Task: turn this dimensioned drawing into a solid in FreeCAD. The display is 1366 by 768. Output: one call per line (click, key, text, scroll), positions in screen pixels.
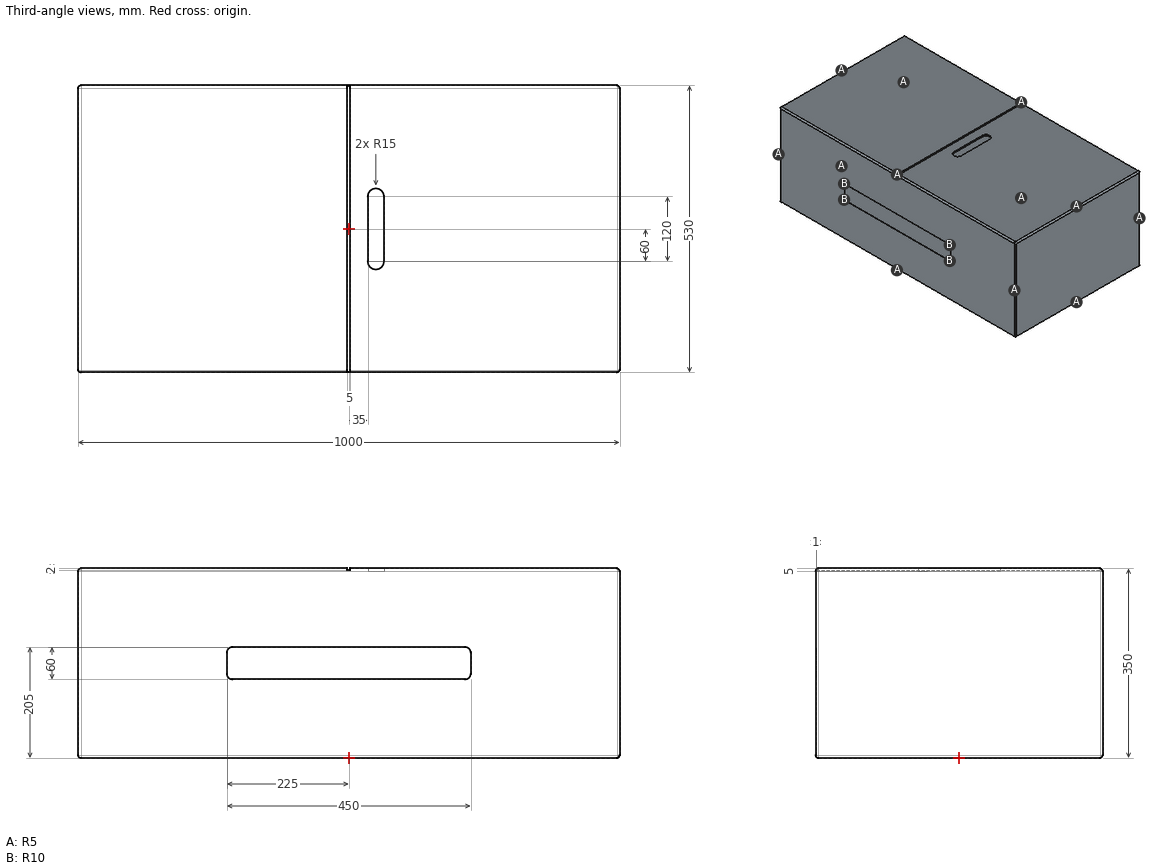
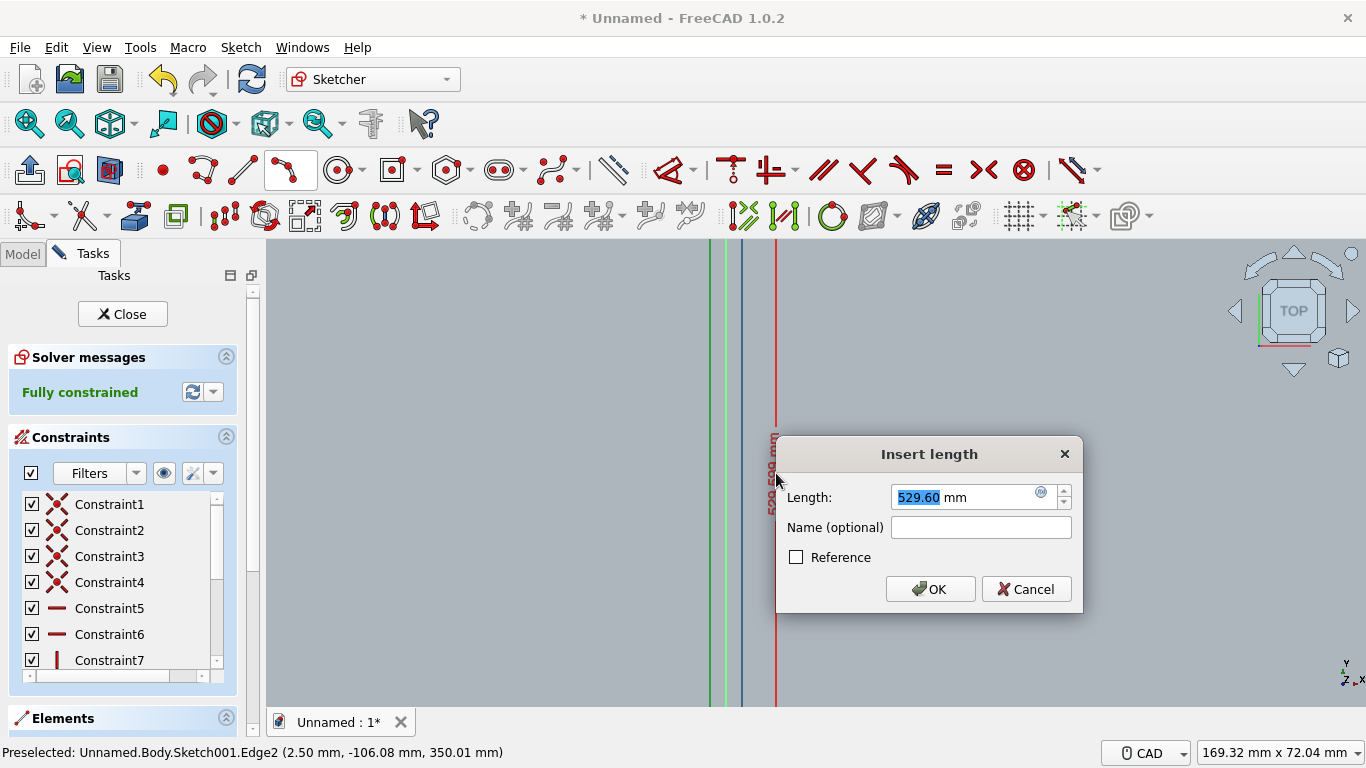
text(530)
key(Return)
key(Escape)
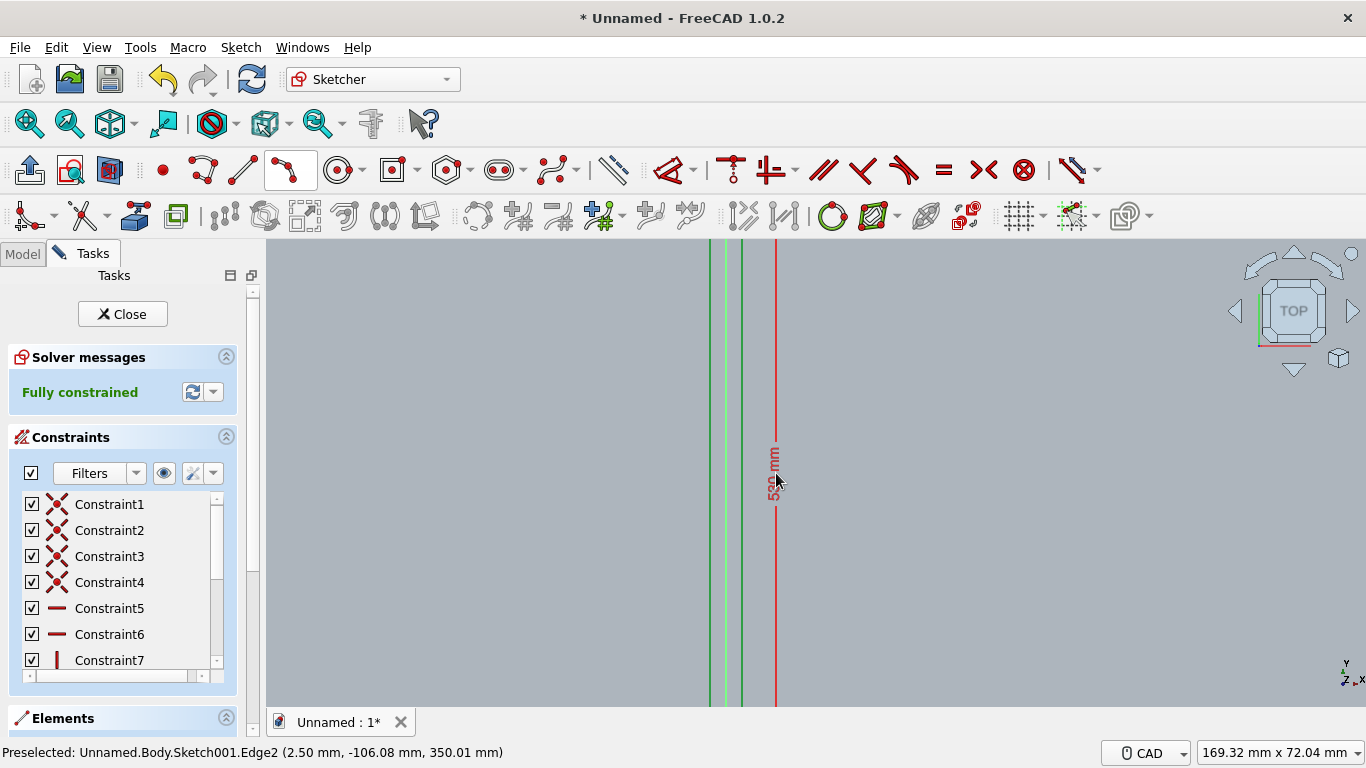
click(123, 314)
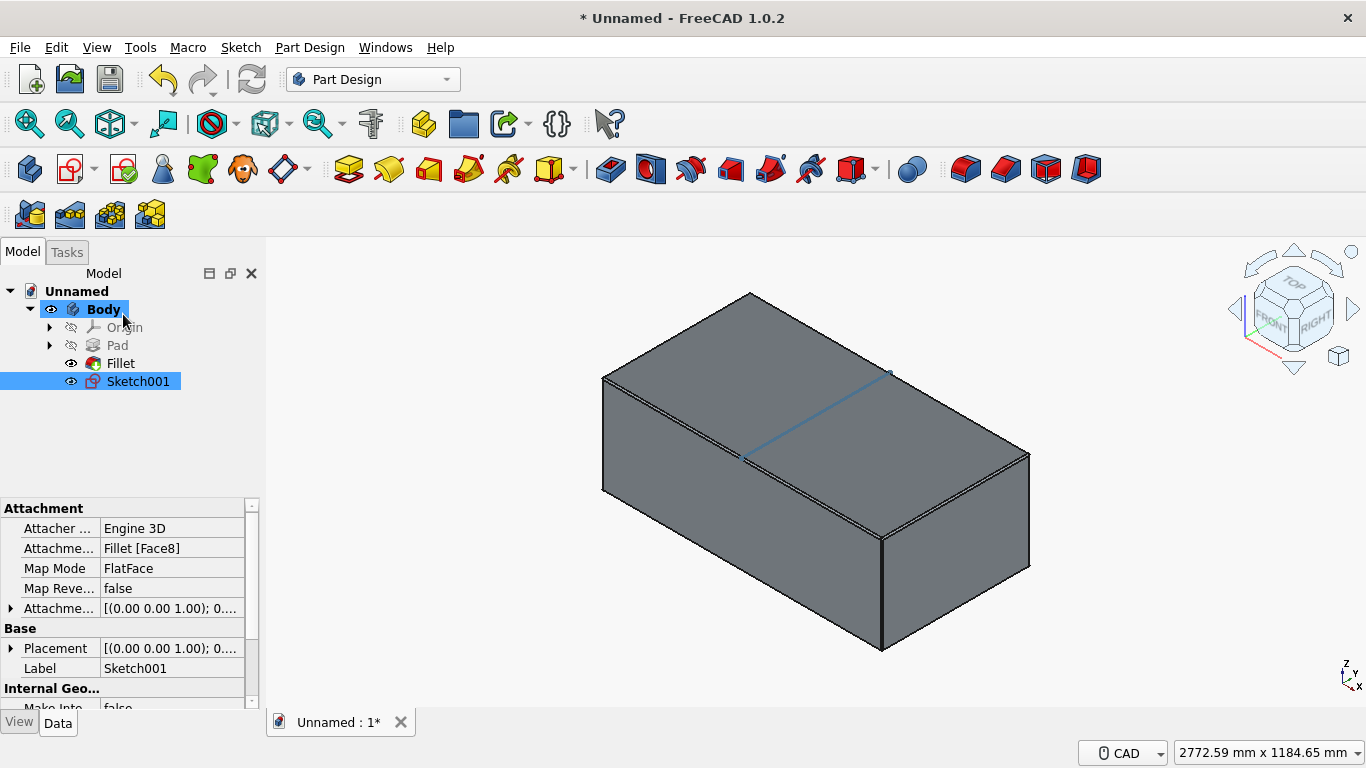
click(612, 170)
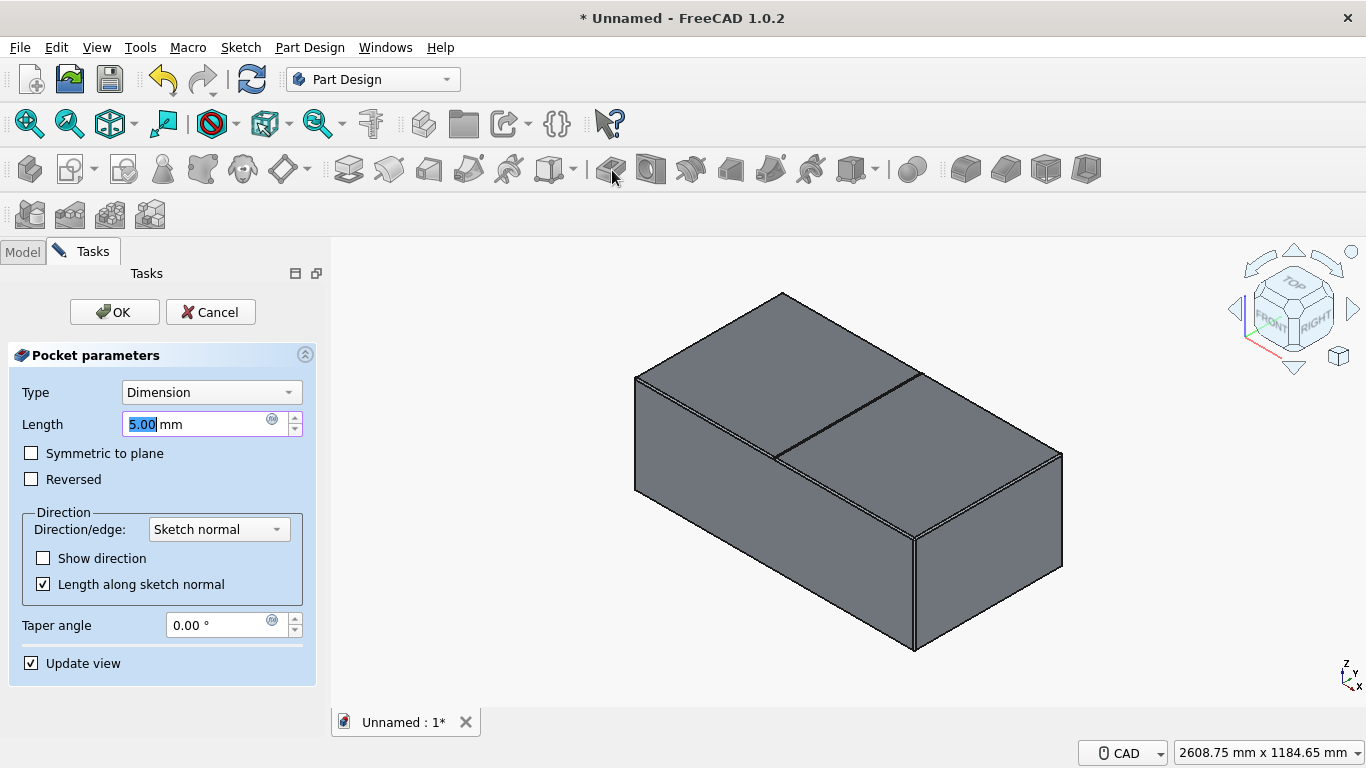
text(2)
key(Tab)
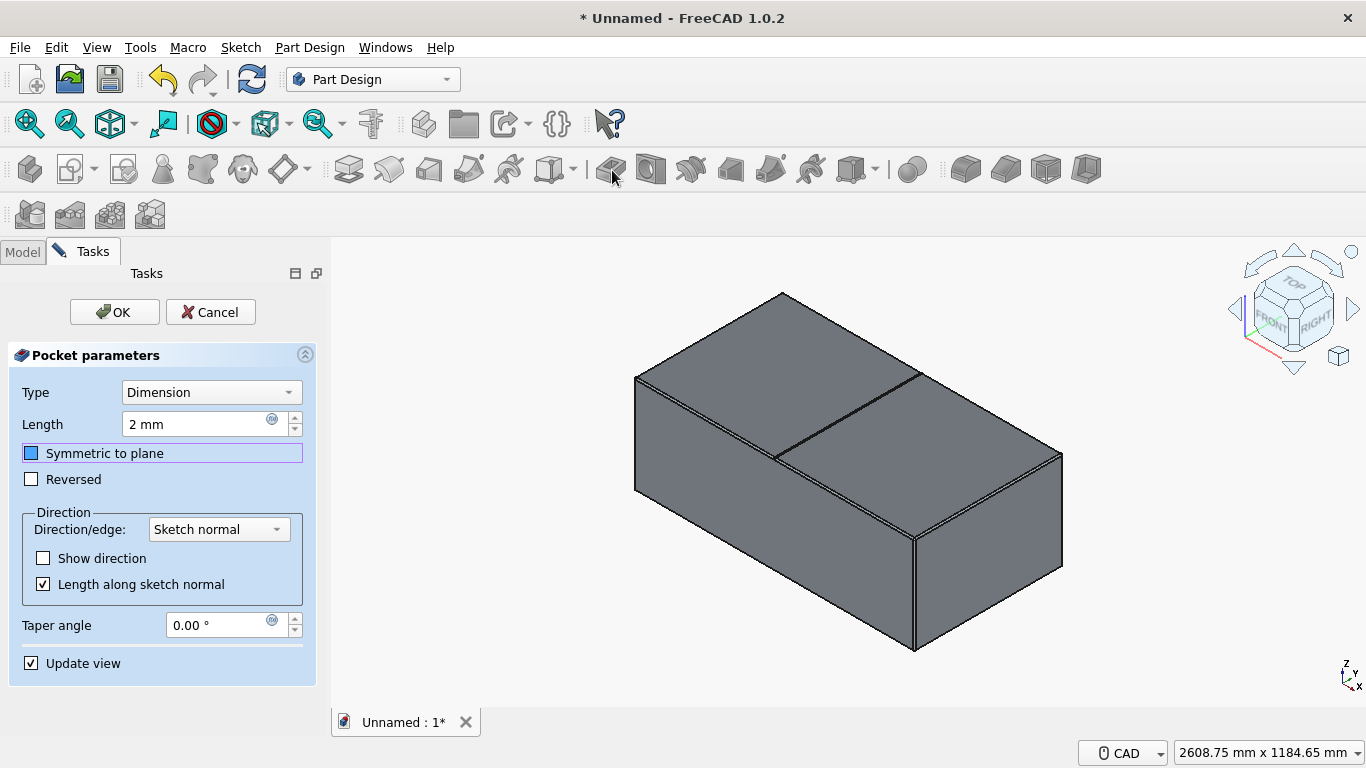
click(115, 312)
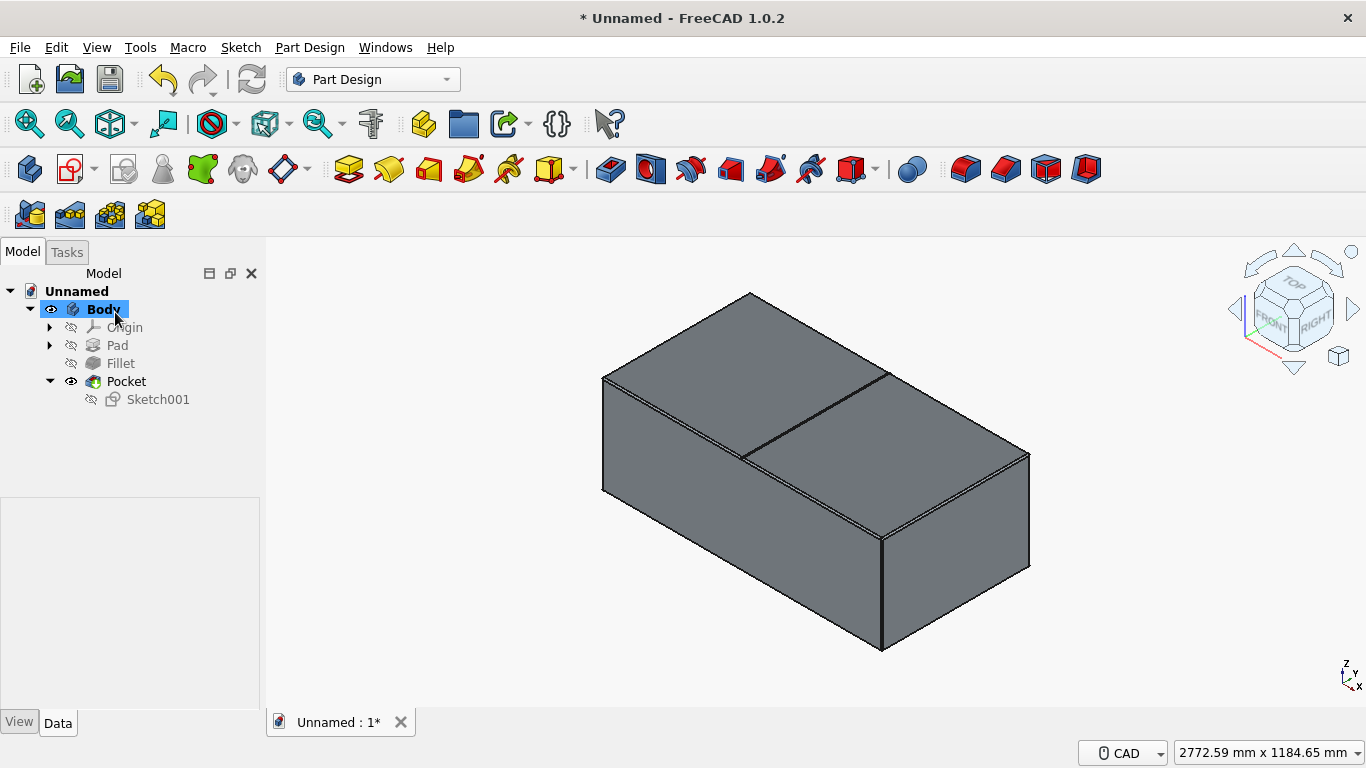
click(886, 455)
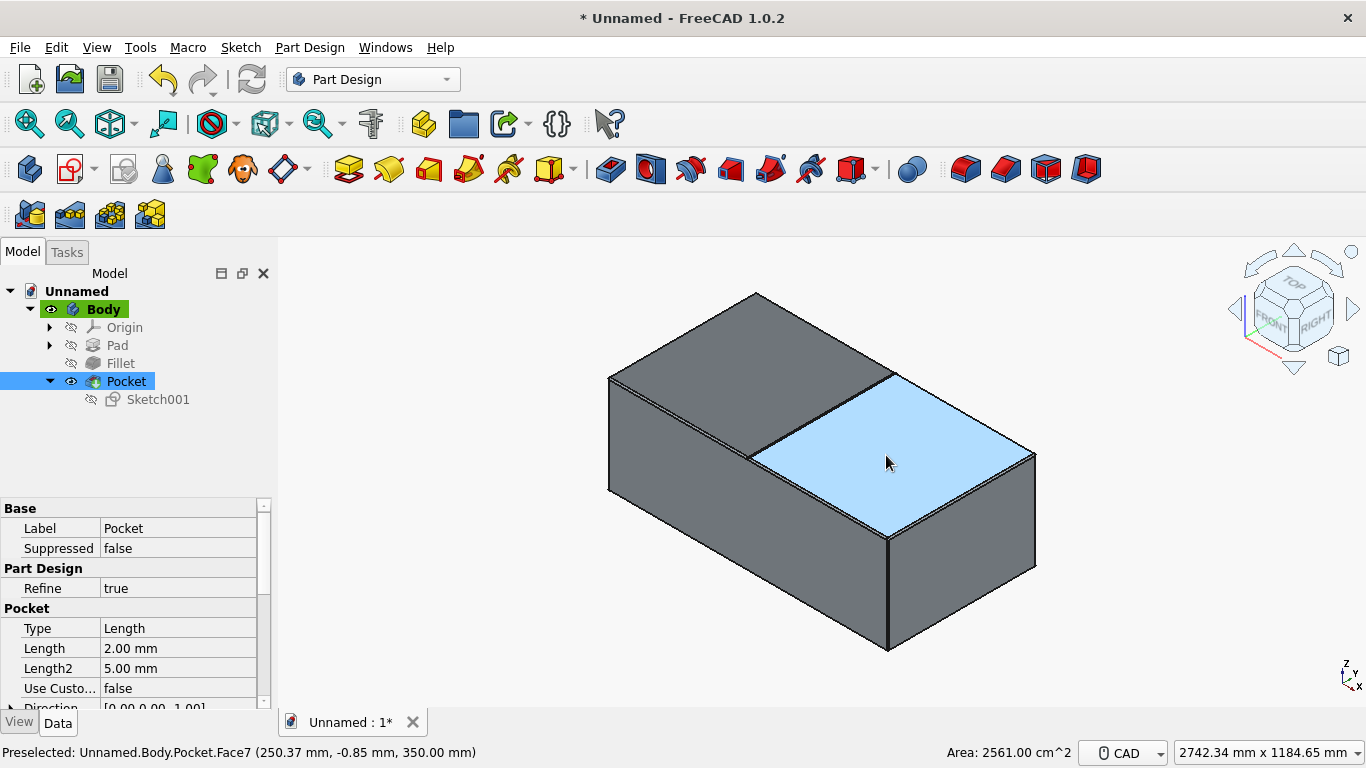
click(70, 170)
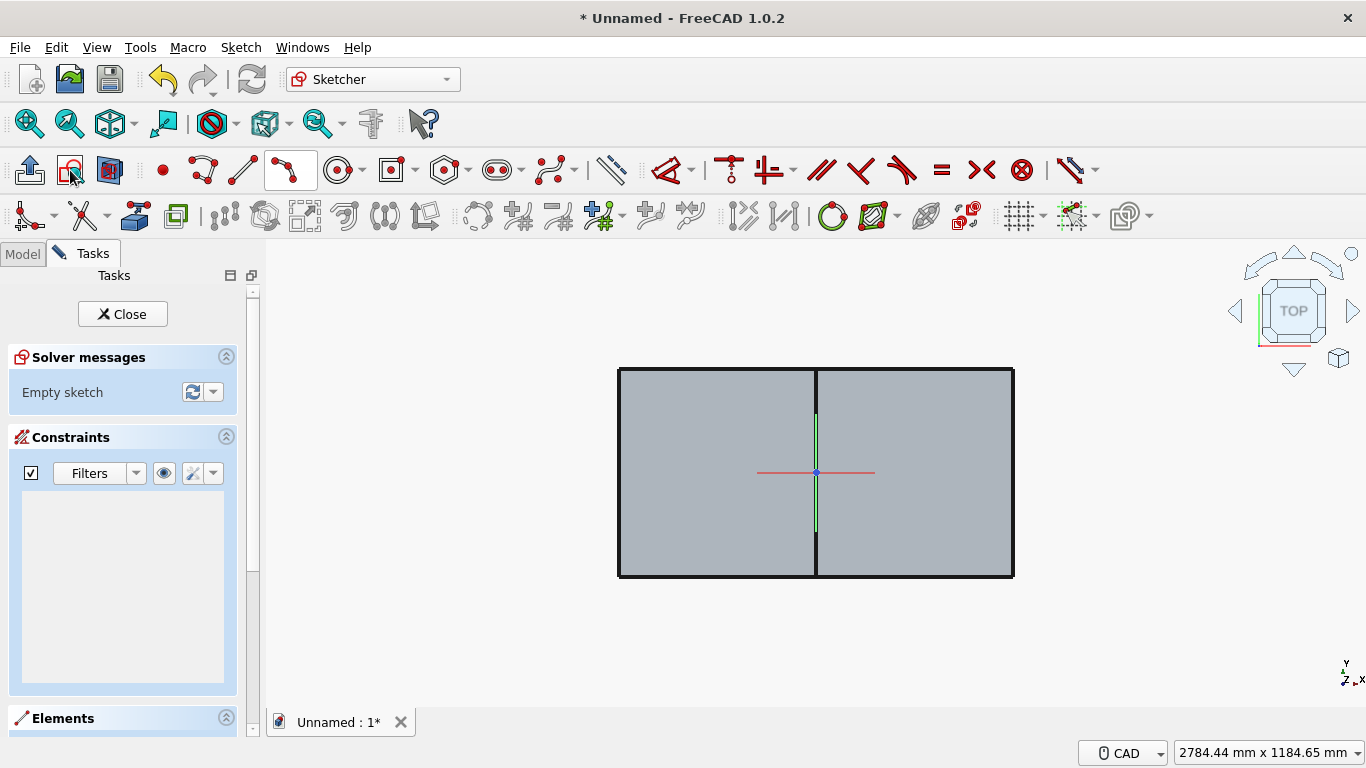
scroll(849, 473, up, 8)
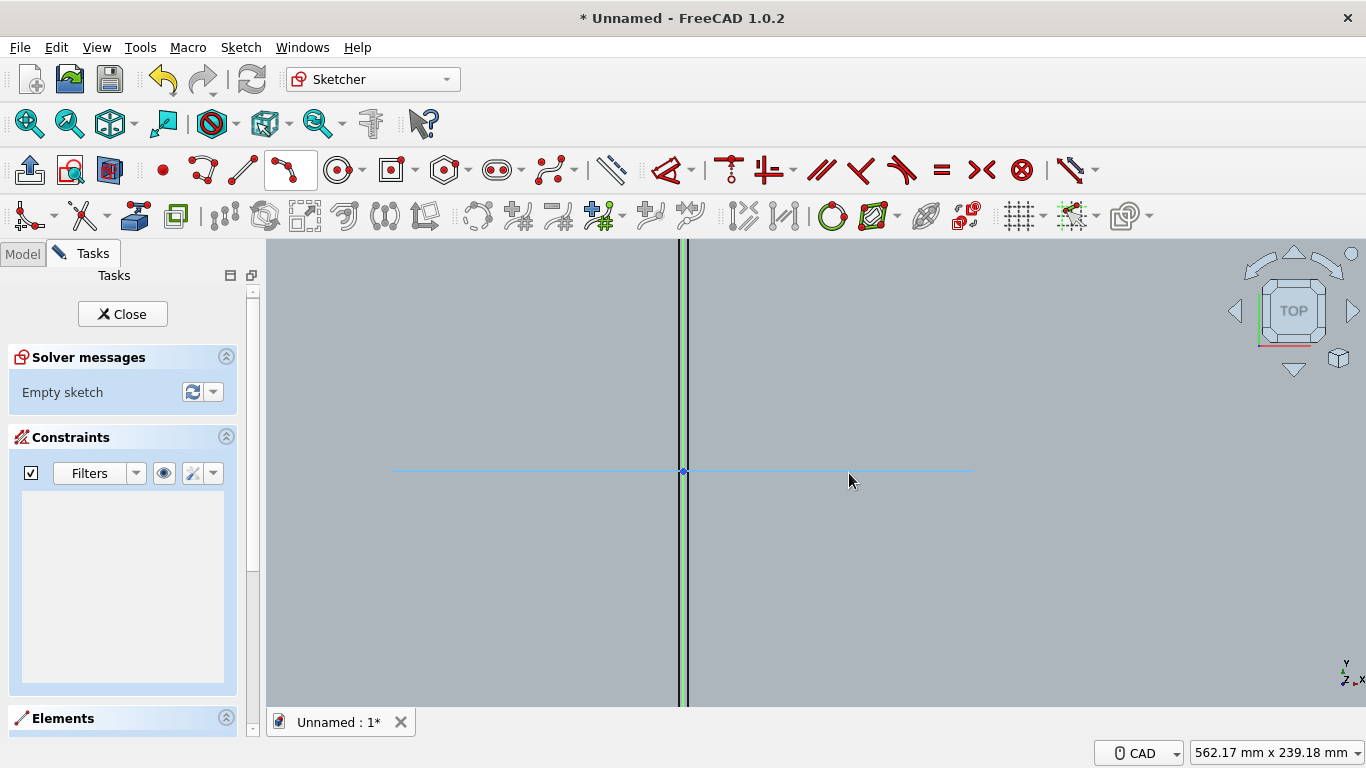
click(498, 170)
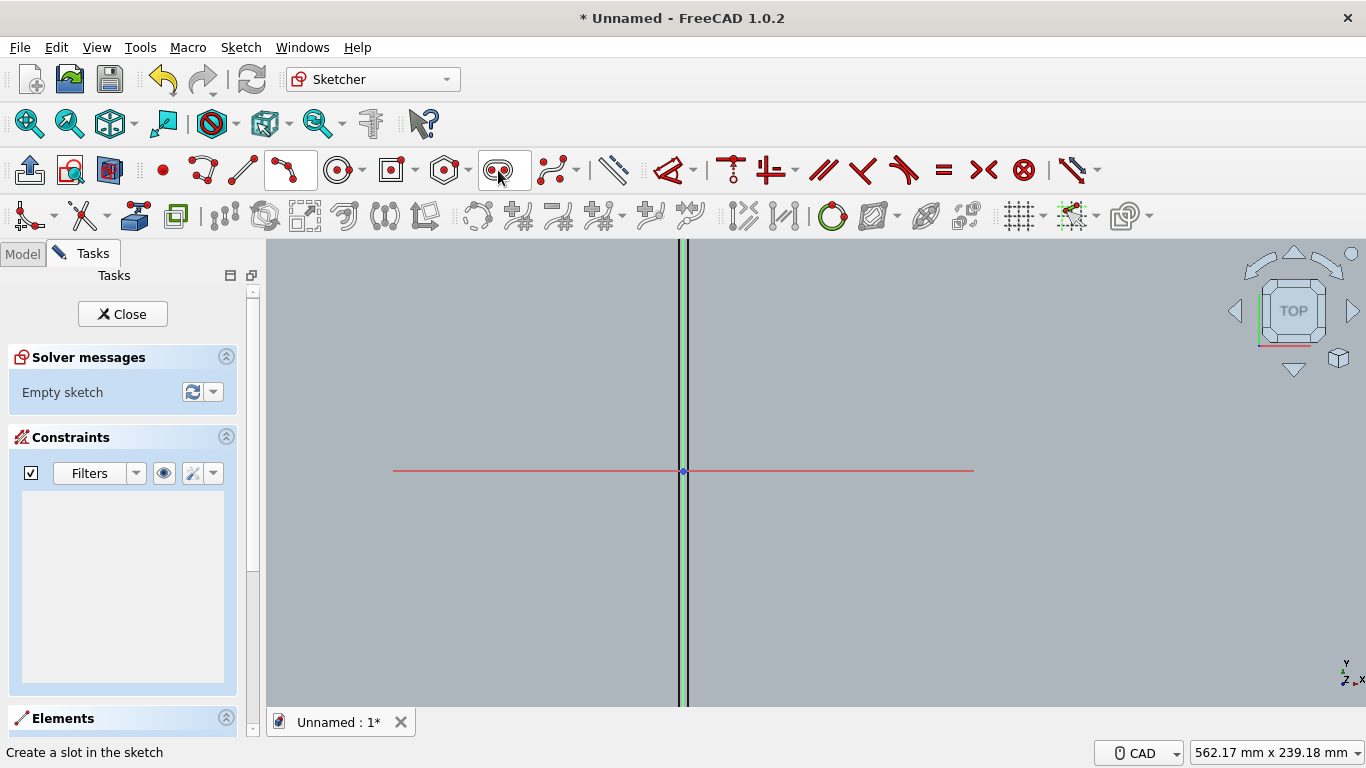
click(781, 588)